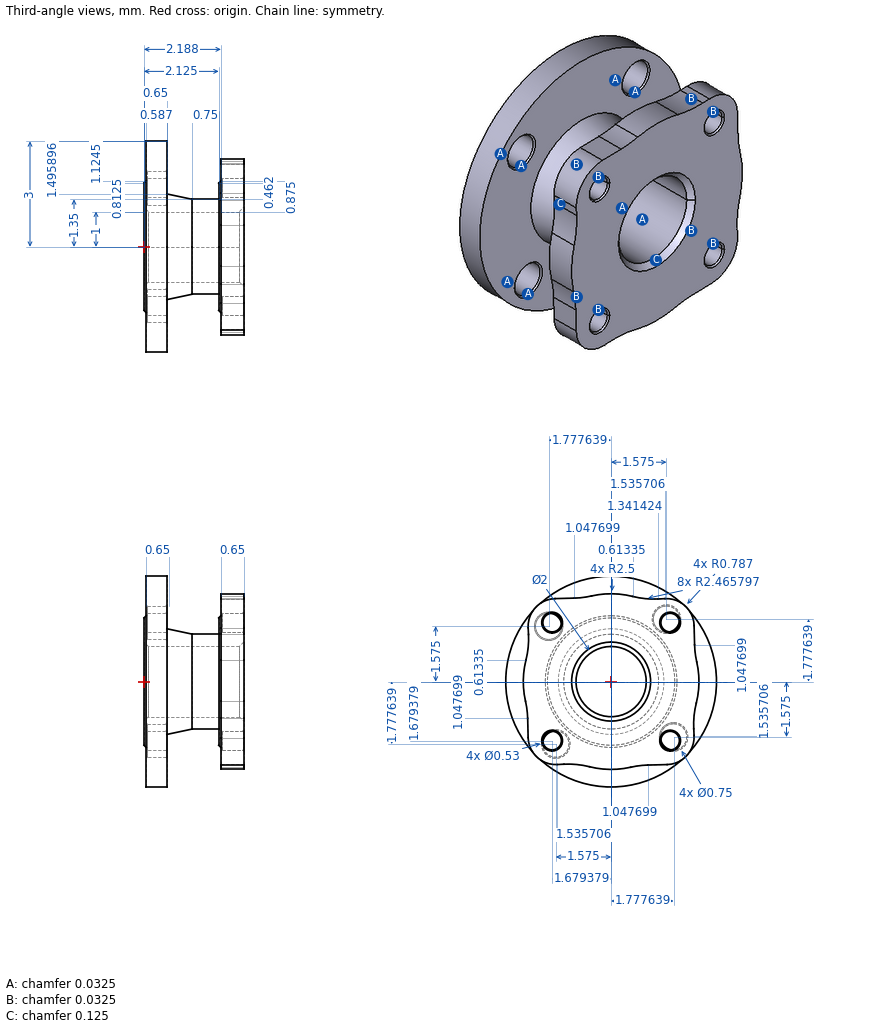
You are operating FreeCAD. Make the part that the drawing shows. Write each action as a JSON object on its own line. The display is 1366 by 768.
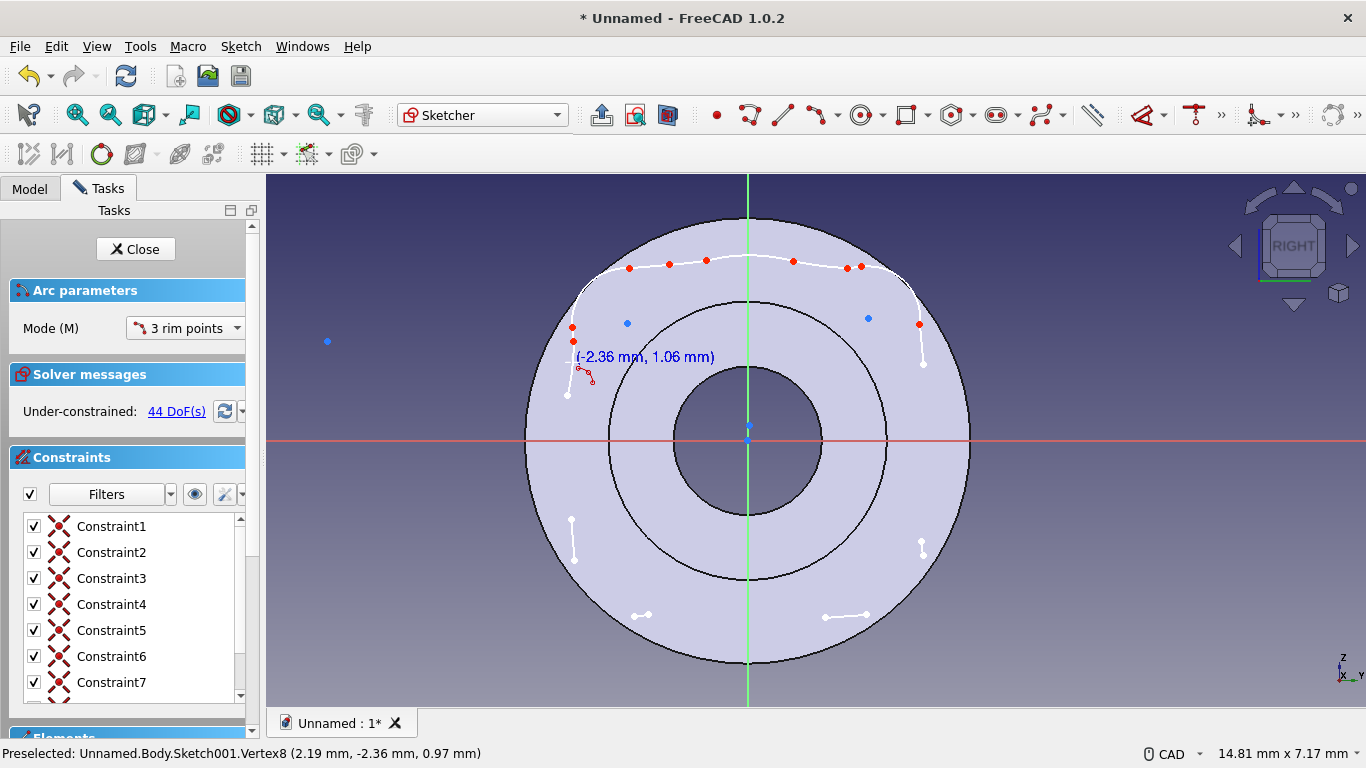
{"action": "left_click", "coordinate": [568, 396]}
{"action": "left_click", "coordinate": [567, 482]}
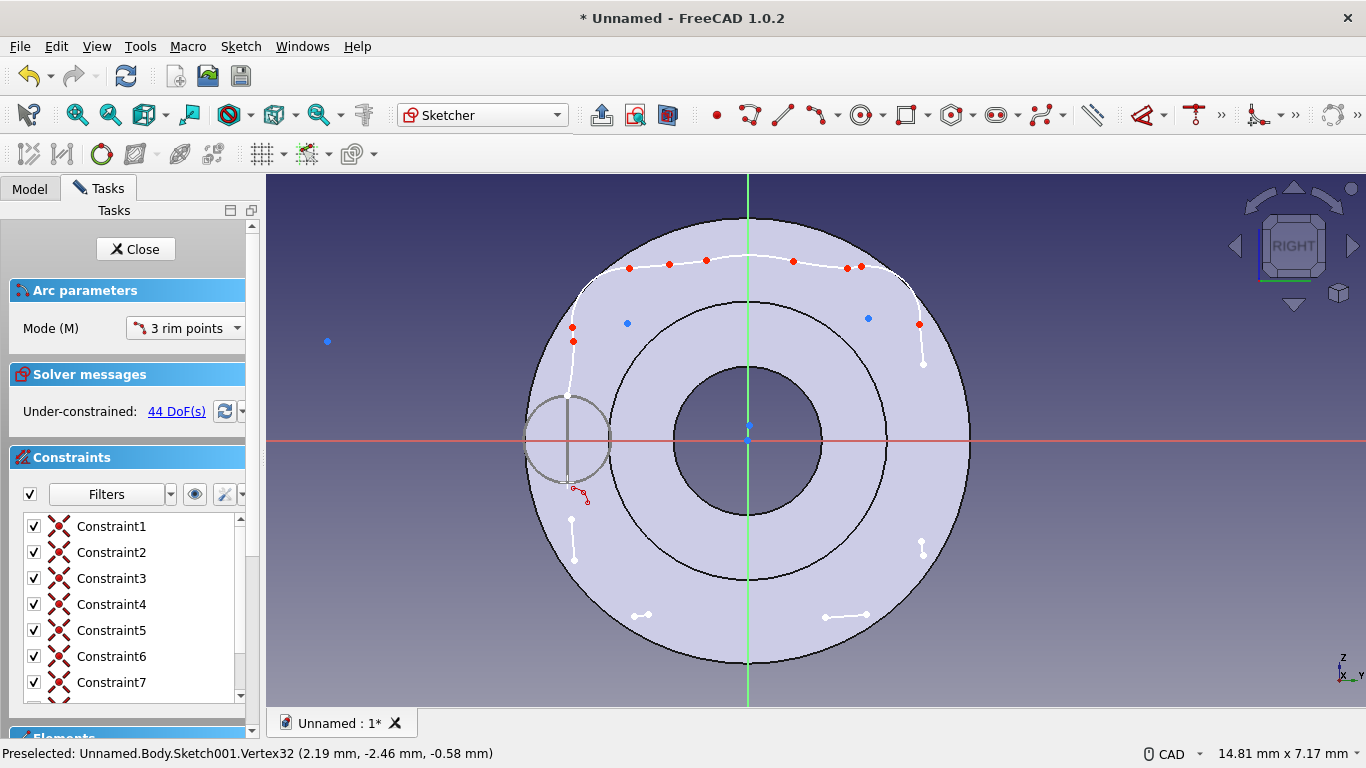
{"action": "scroll", "coordinate": [562, 448], "scroll_direction": "up", "scroll_amount": 6}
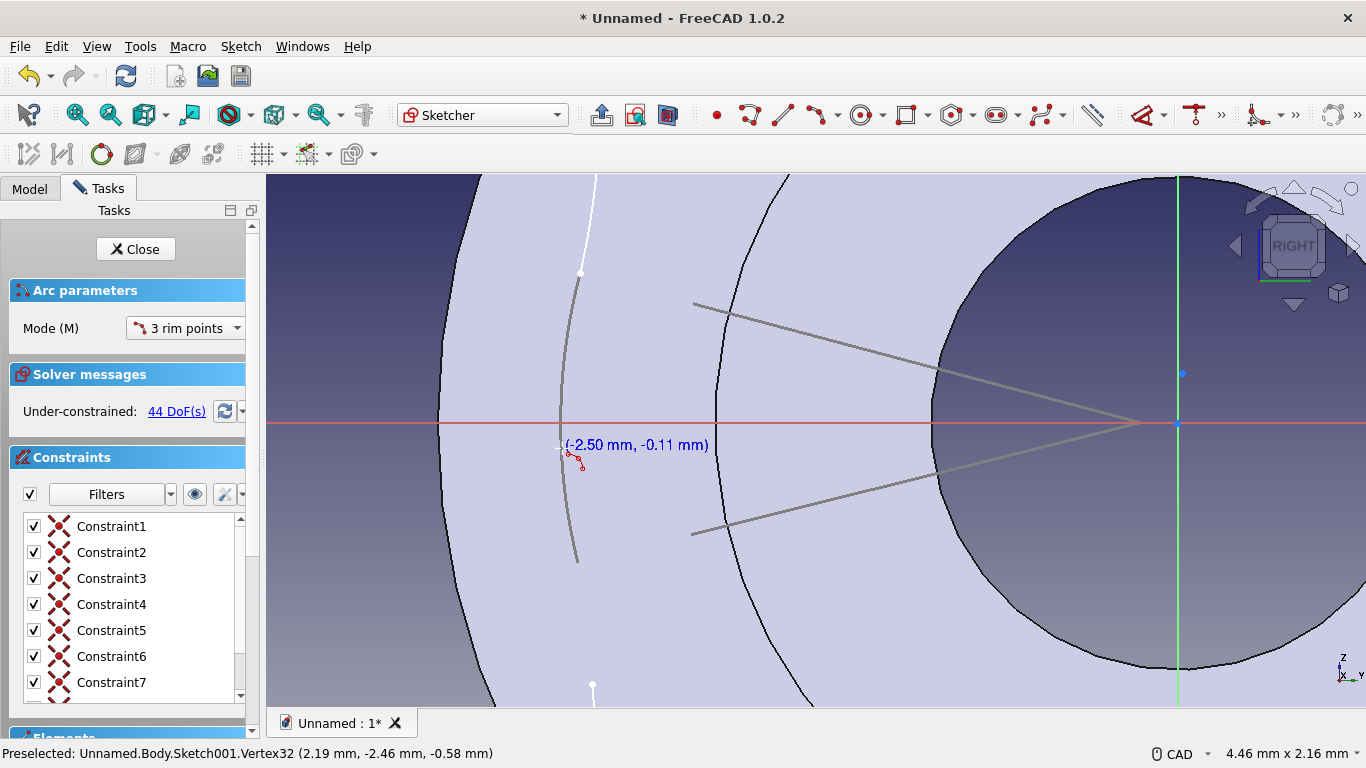
{"action": "left_click", "coordinate": [561, 445]}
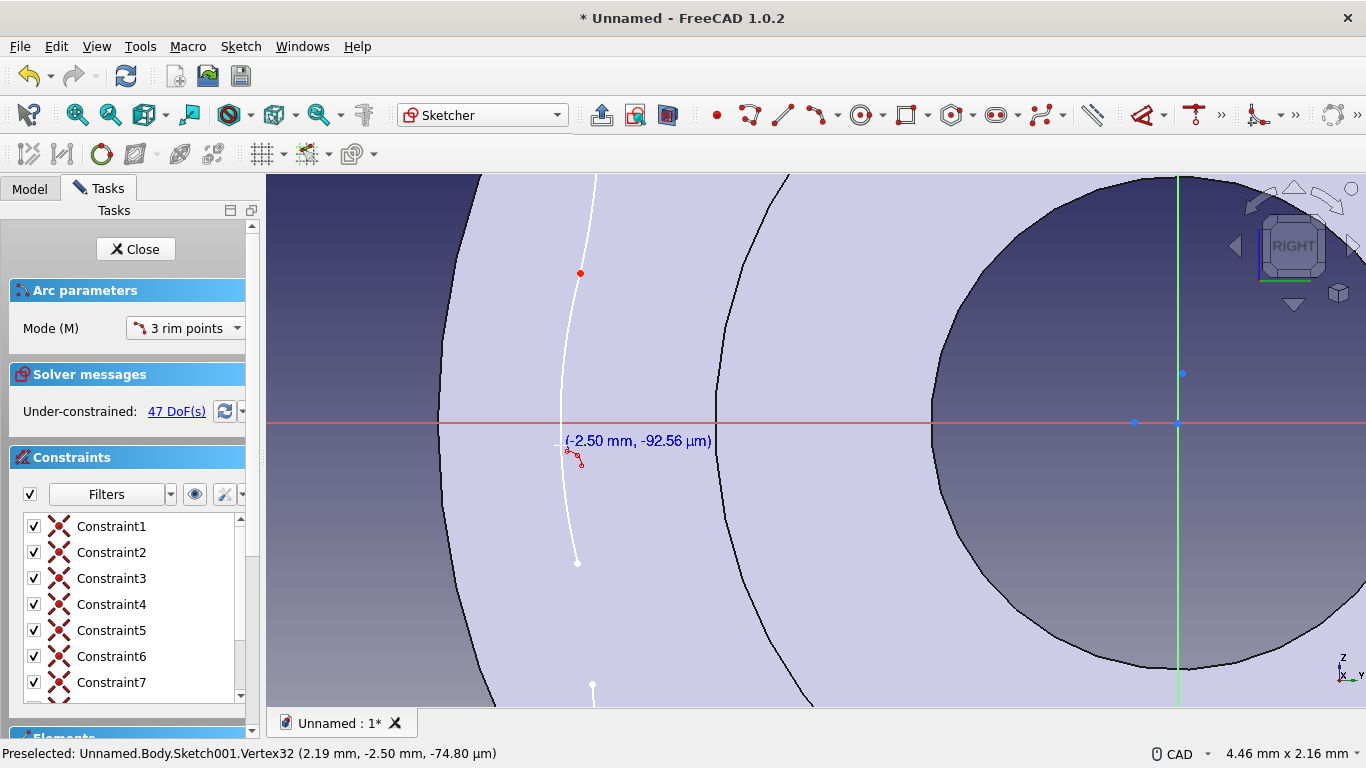
{"action": "scroll", "coordinate": [562, 448], "scroll_direction": "down", "scroll_amount": 6}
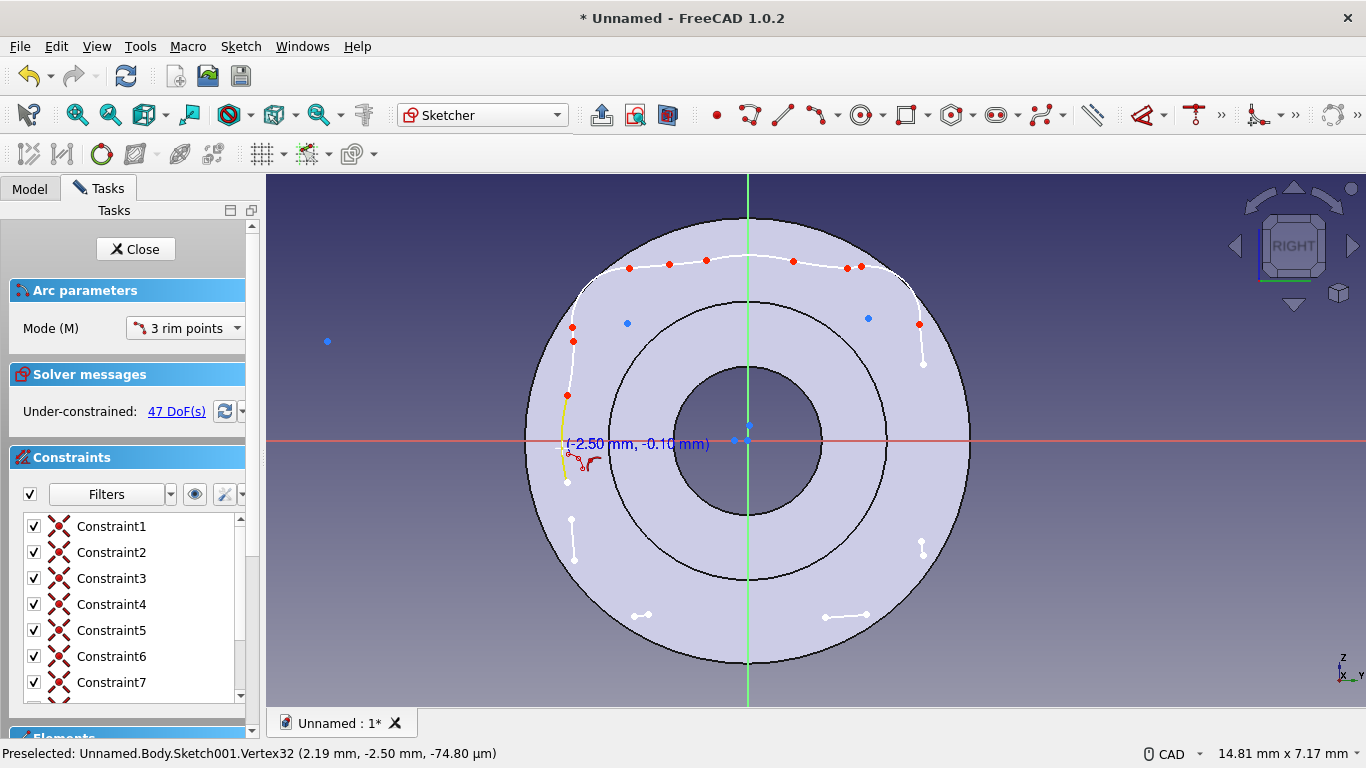
{"action": "left_click", "coordinate": [567, 483]}
{"action": "left_click", "coordinate": [571, 520]}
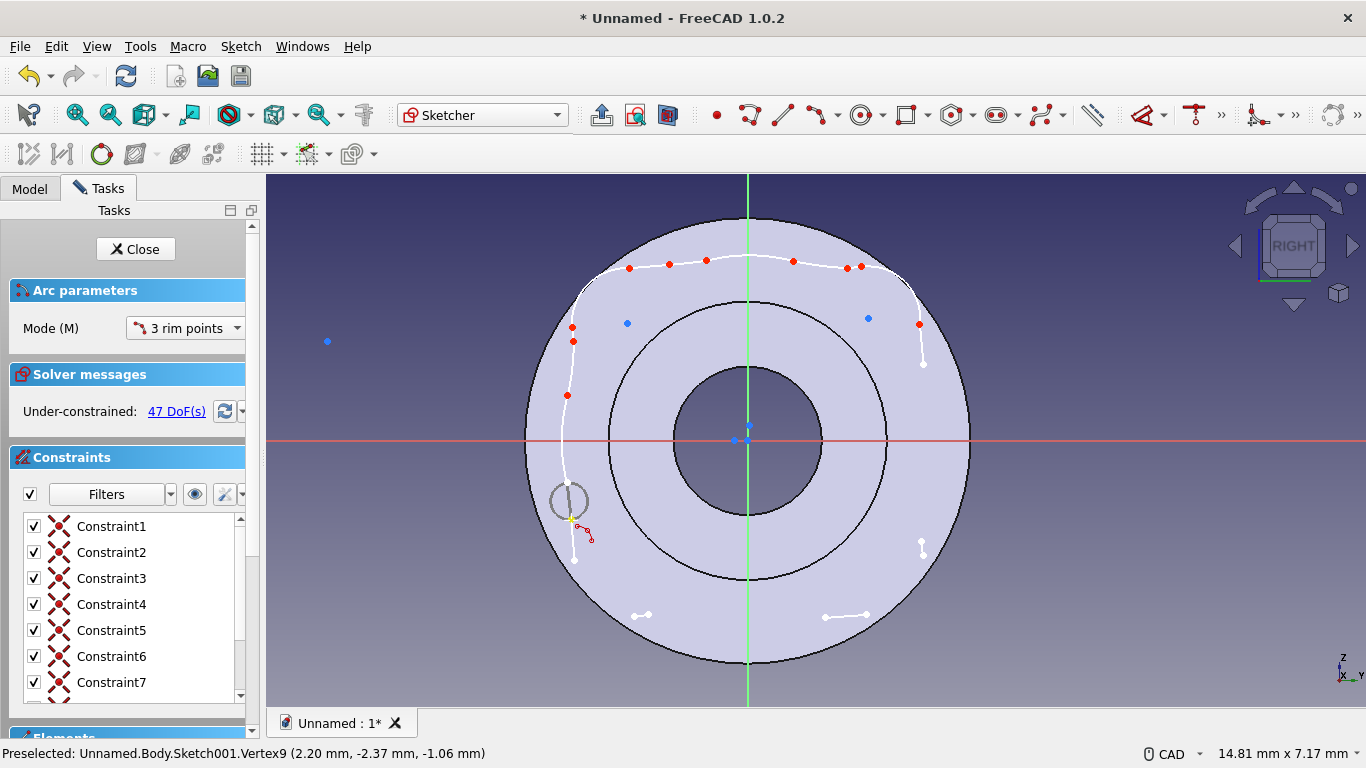
{"action": "scroll", "coordinate": [570, 500], "scroll_direction": "up", "scroll_amount": 15}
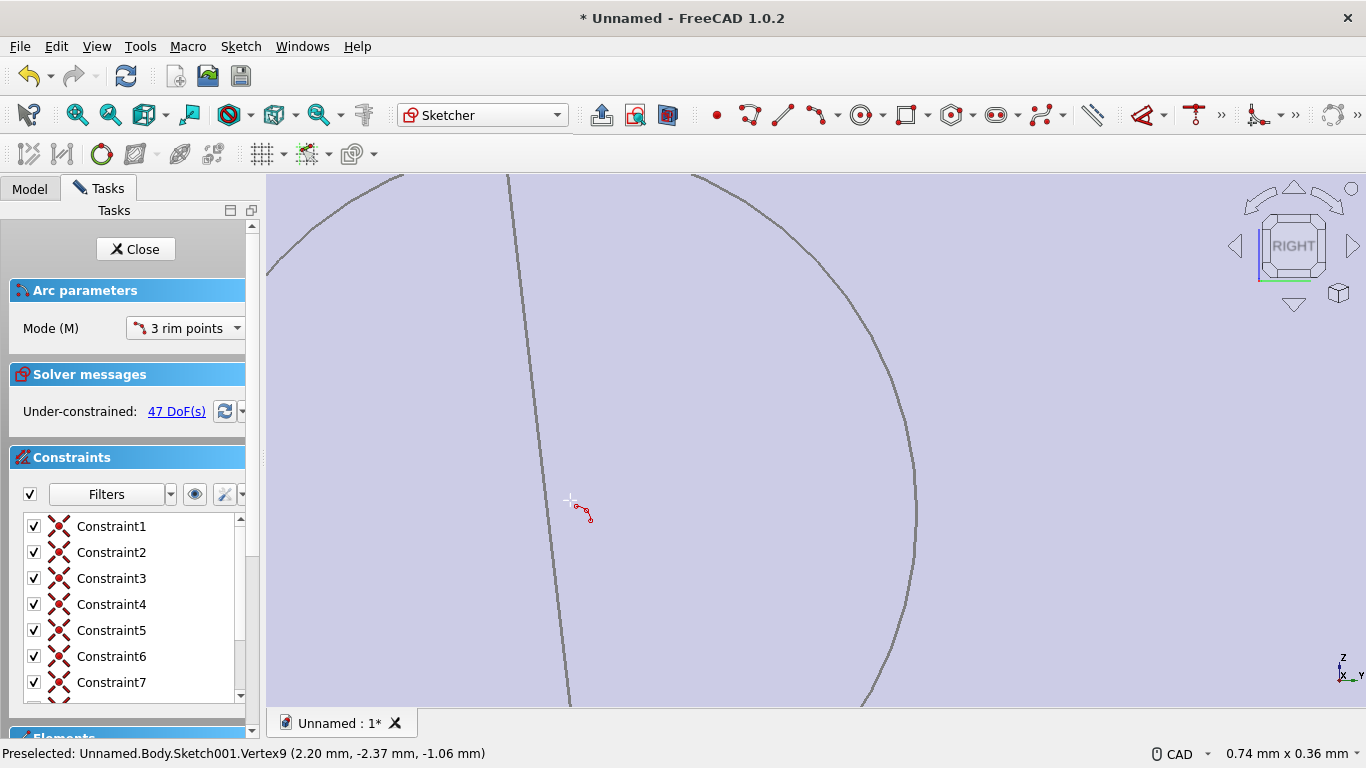
{"action": "left_click", "coordinate": [561, 497]}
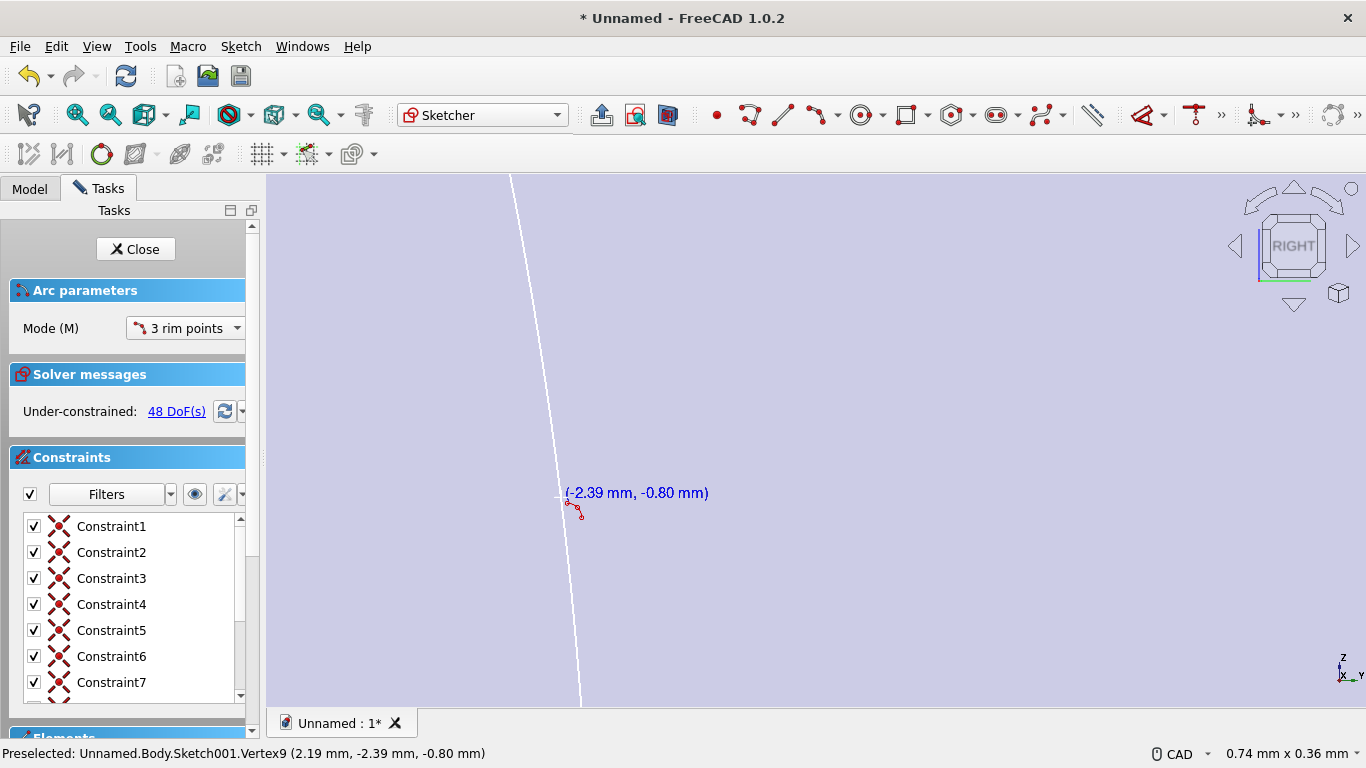
{"action": "scroll", "coordinate": [570, 500], "scroll_direction": "down", "scroll_amount": 15}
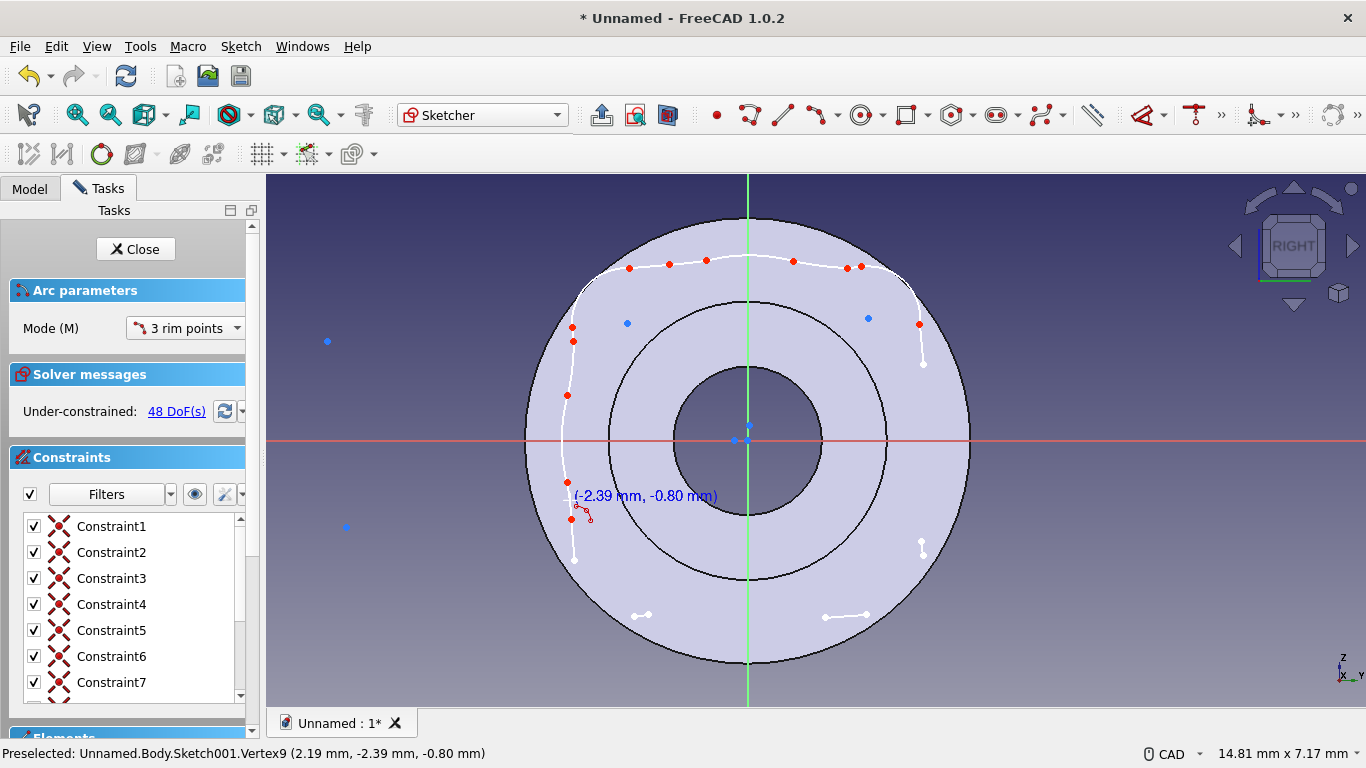
{"action": "left_click", "coordinate": [575, 560]}